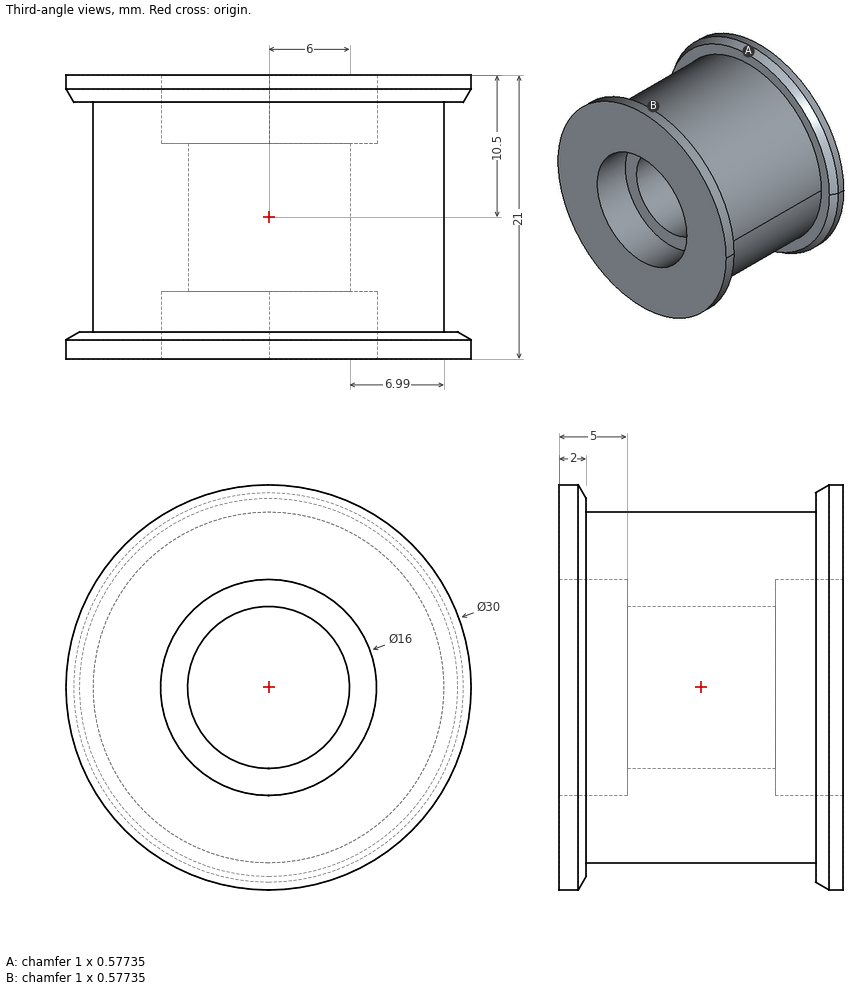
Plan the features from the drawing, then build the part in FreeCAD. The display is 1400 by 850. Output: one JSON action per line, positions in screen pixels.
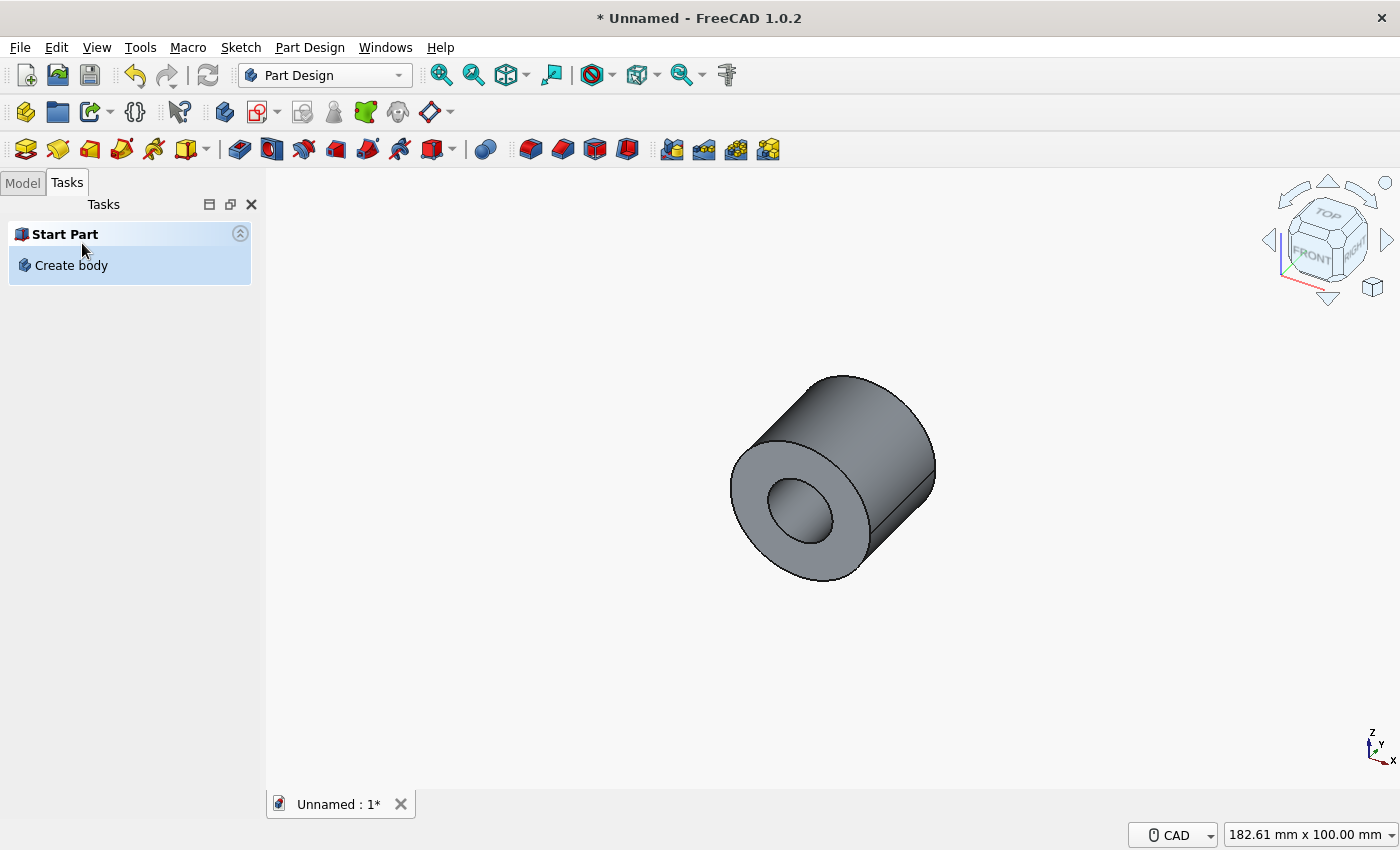
{"action": "left_click", "coordinate": [442, 76]}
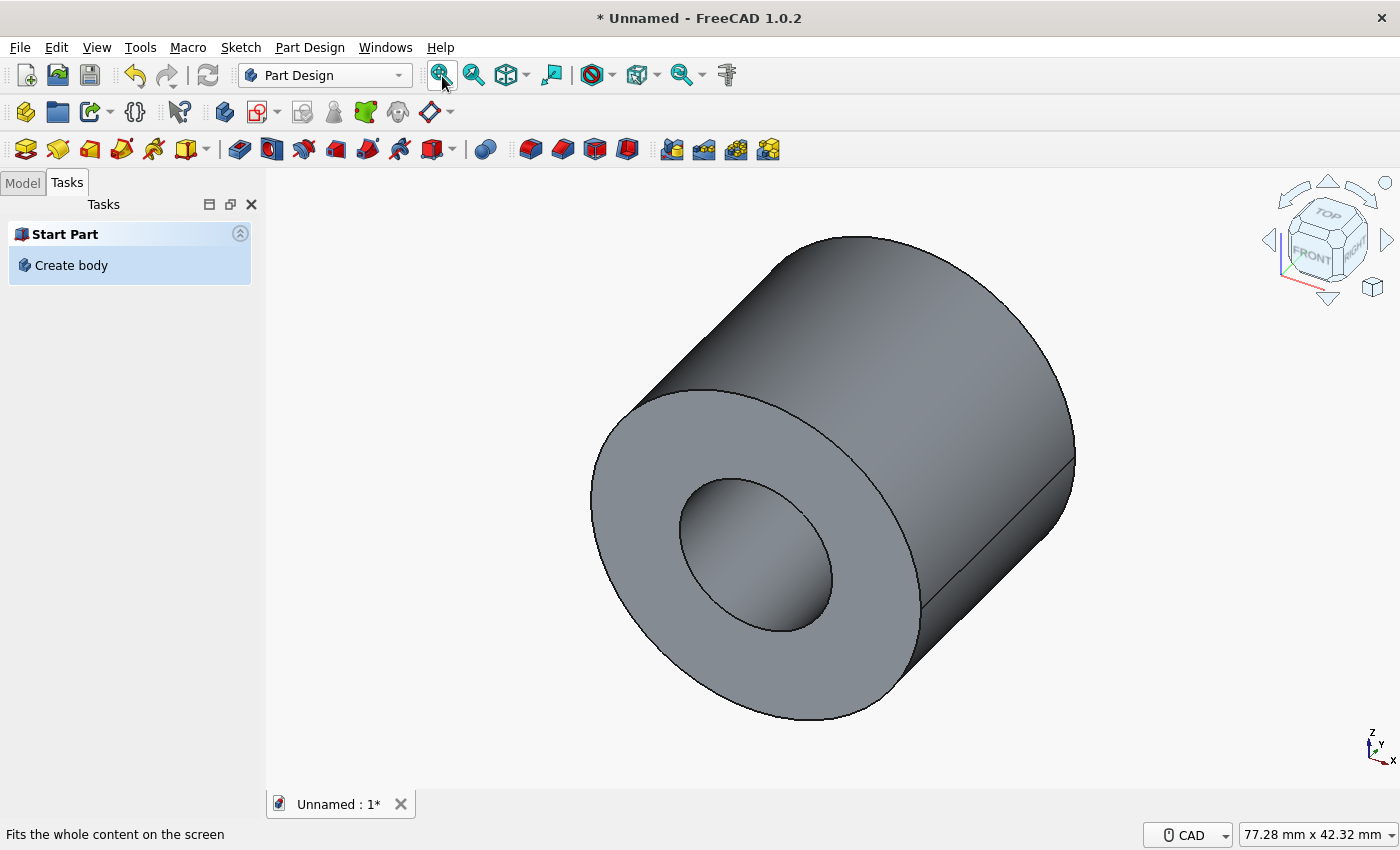
{"action": "left_click", "coordinate": [850, 674]}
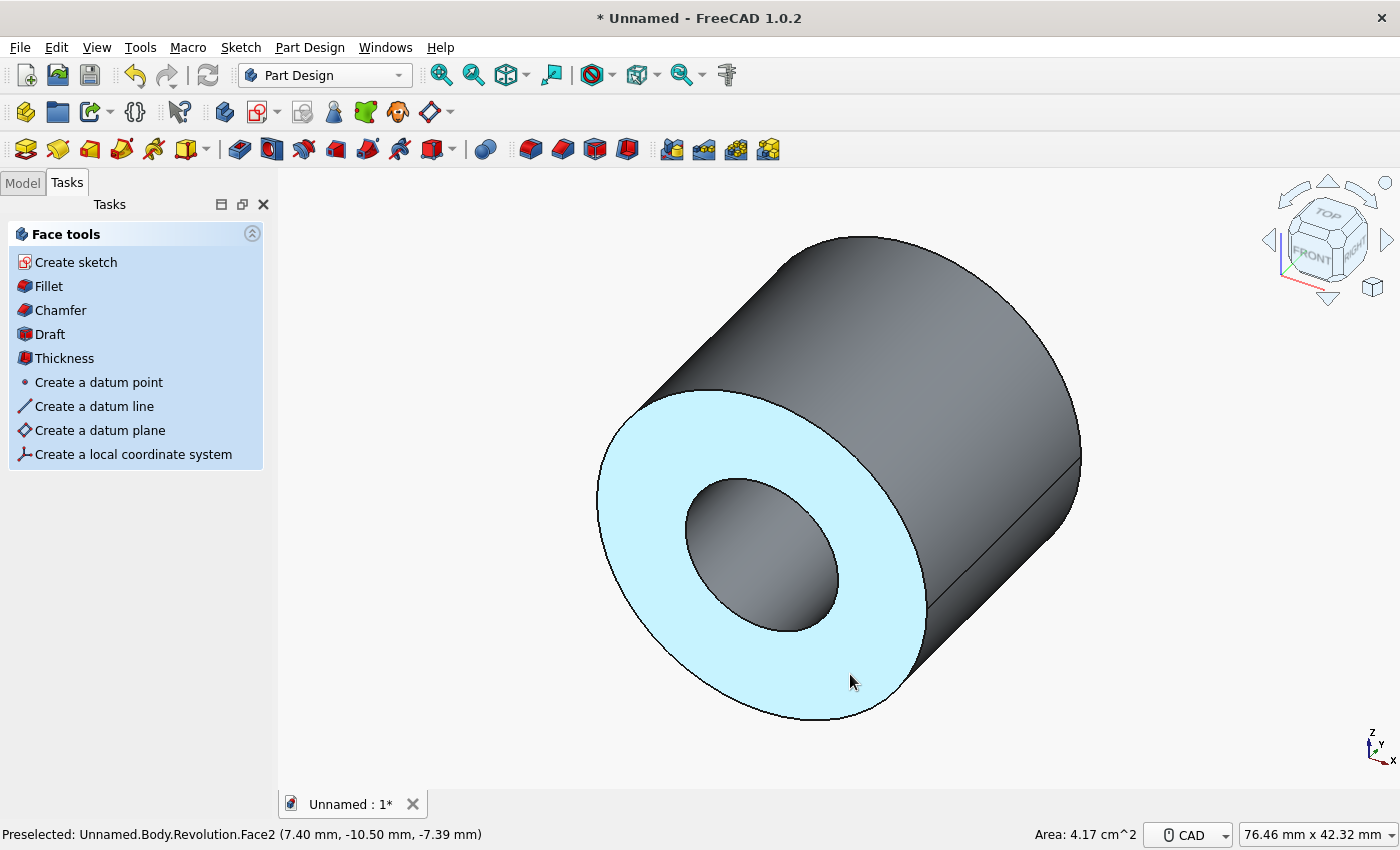
{"action": "left_click", "coordinate": [258, 112]}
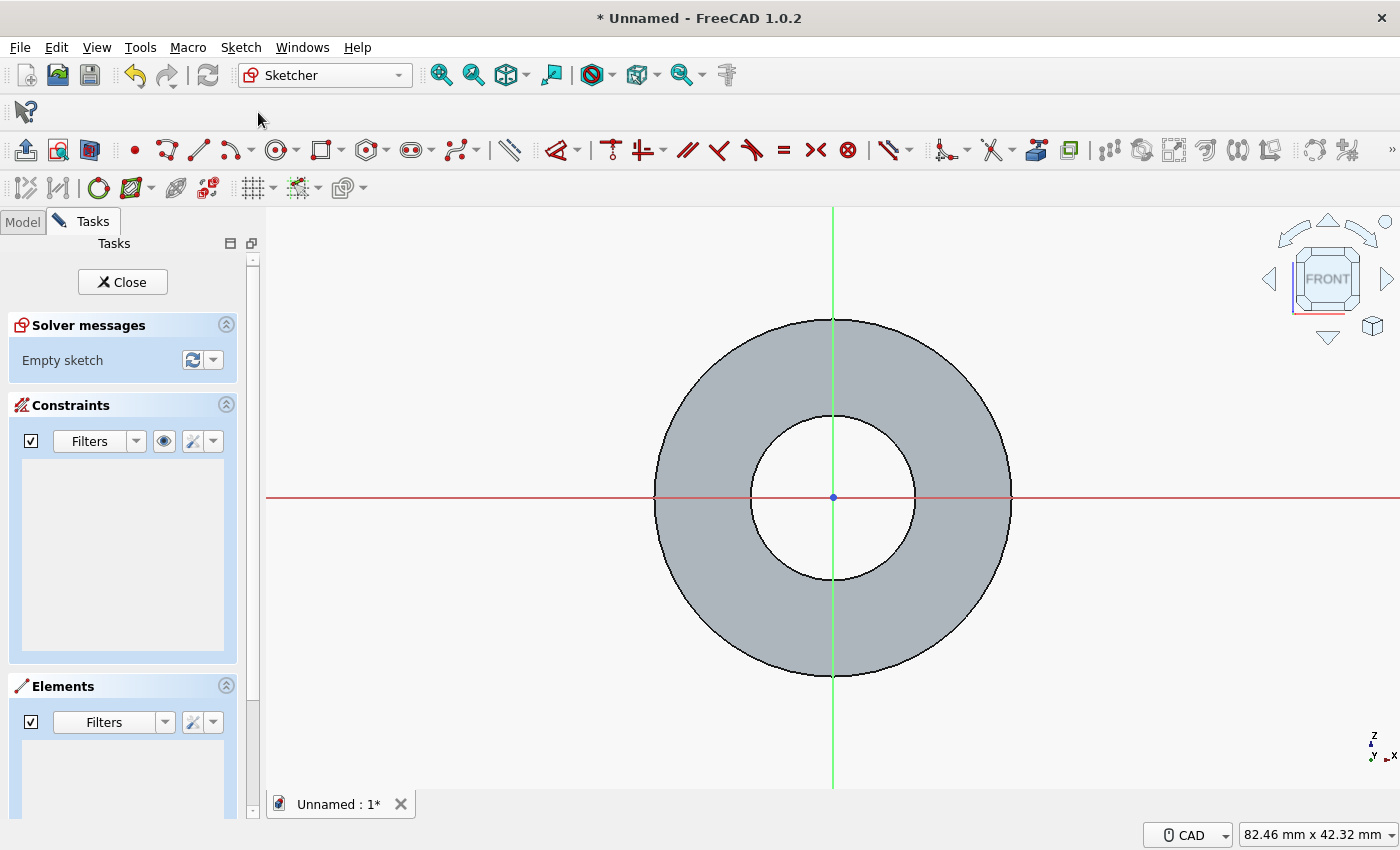
{"action": "scroll", "coordinate": [916, 498], "scroll_direction": "up", "scroll_amount": 3}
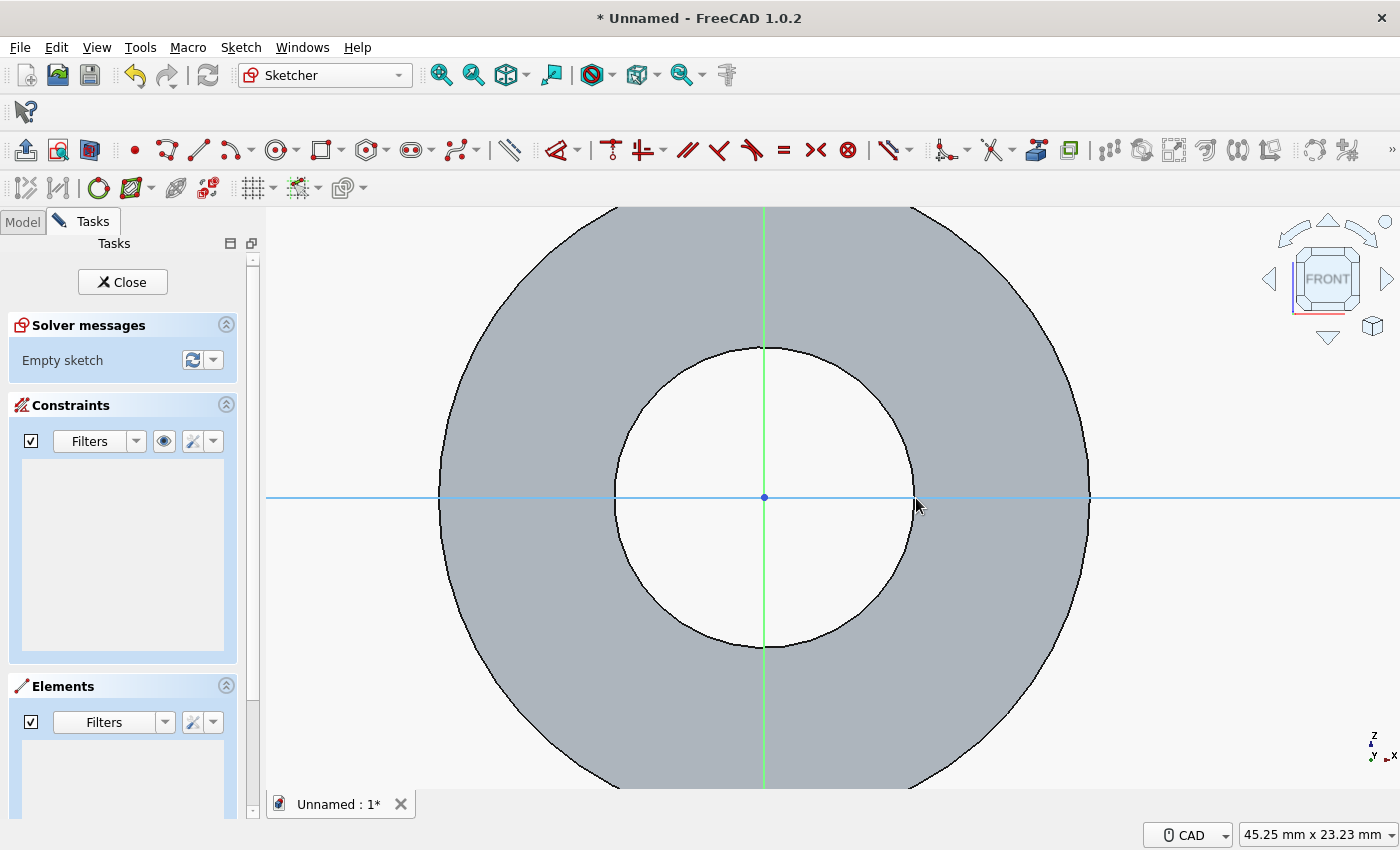
{"action": "left_click", "coordinate": [276, 150]}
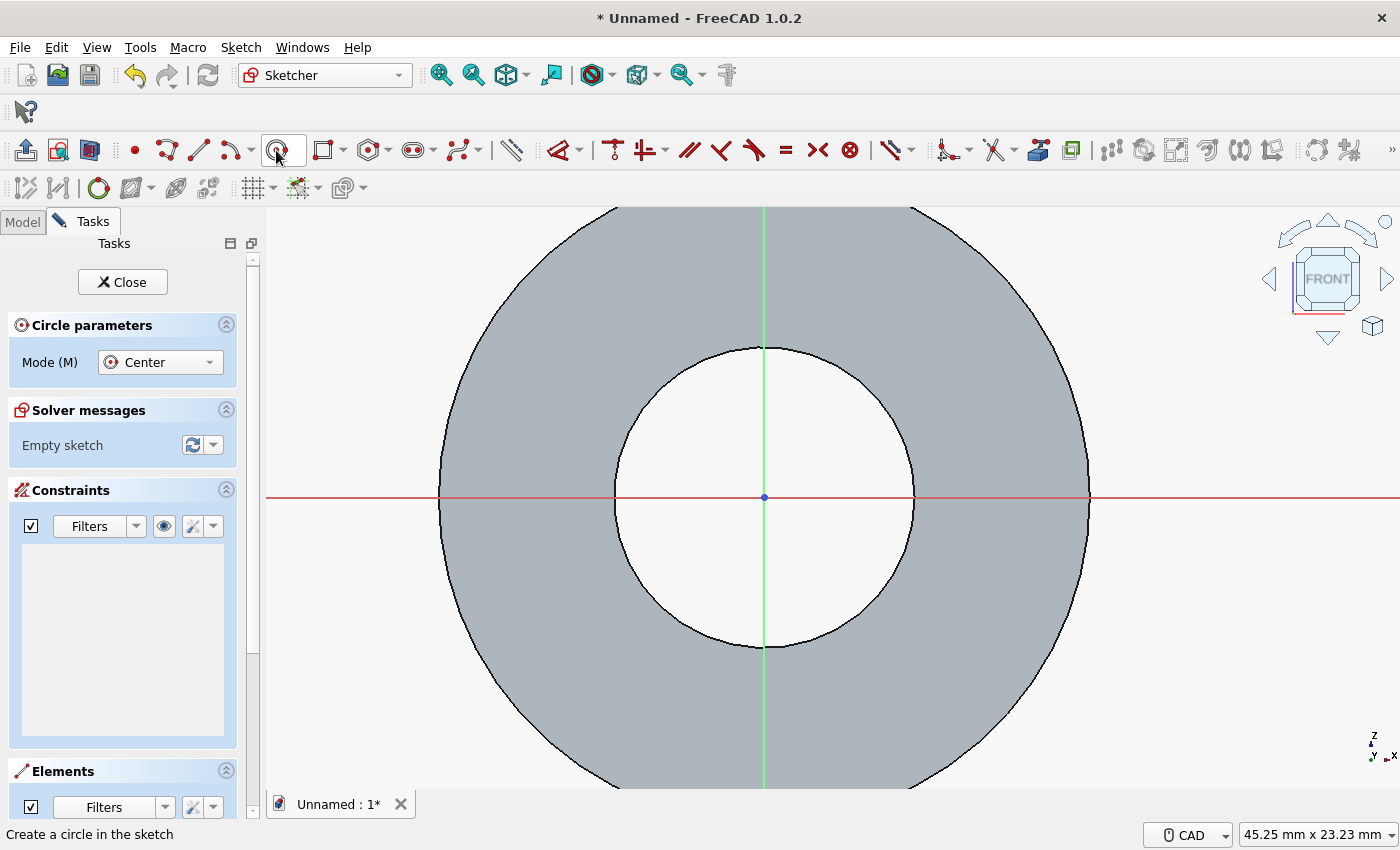
{"action": "left_click", "coordinate": [764, 498]}
{"action": "mouse_move", "coordinate": [906, 356]}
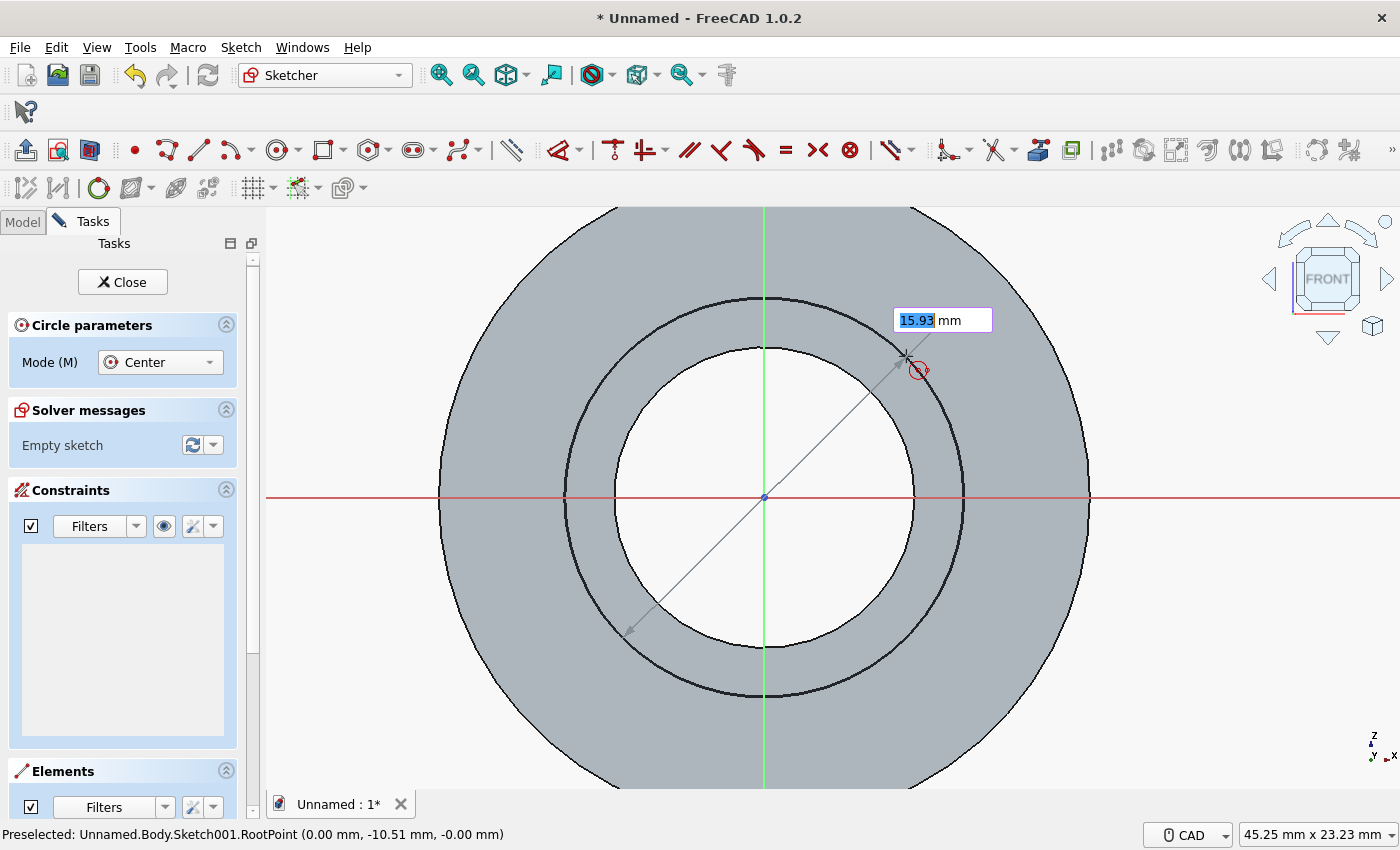
{"action": "type", "text": "16"}
{"action": "key", "text": "Return"}
{"action": "key", "text": "Escape"}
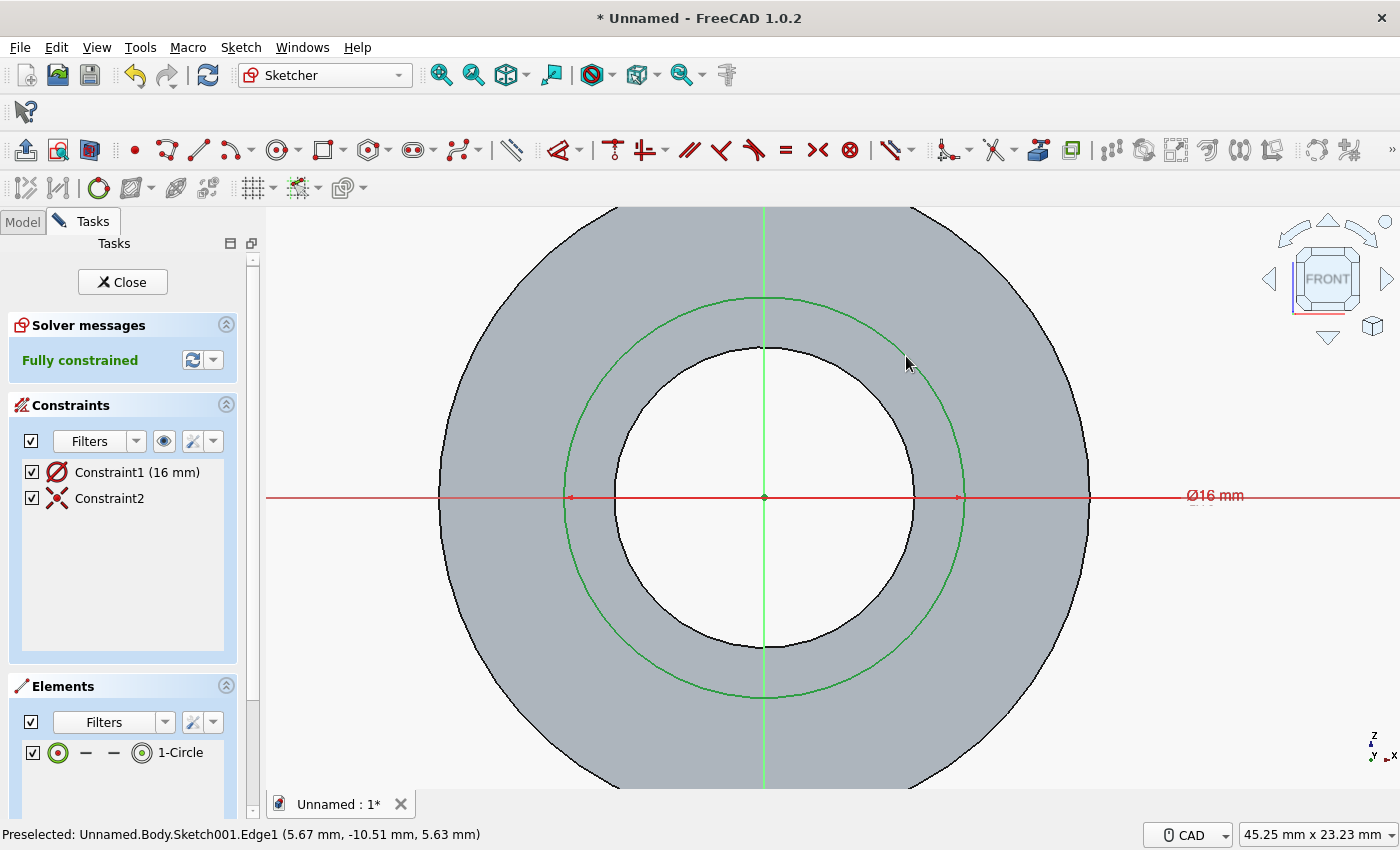
{"action": "left_click", "coordinate": [123, 282]}